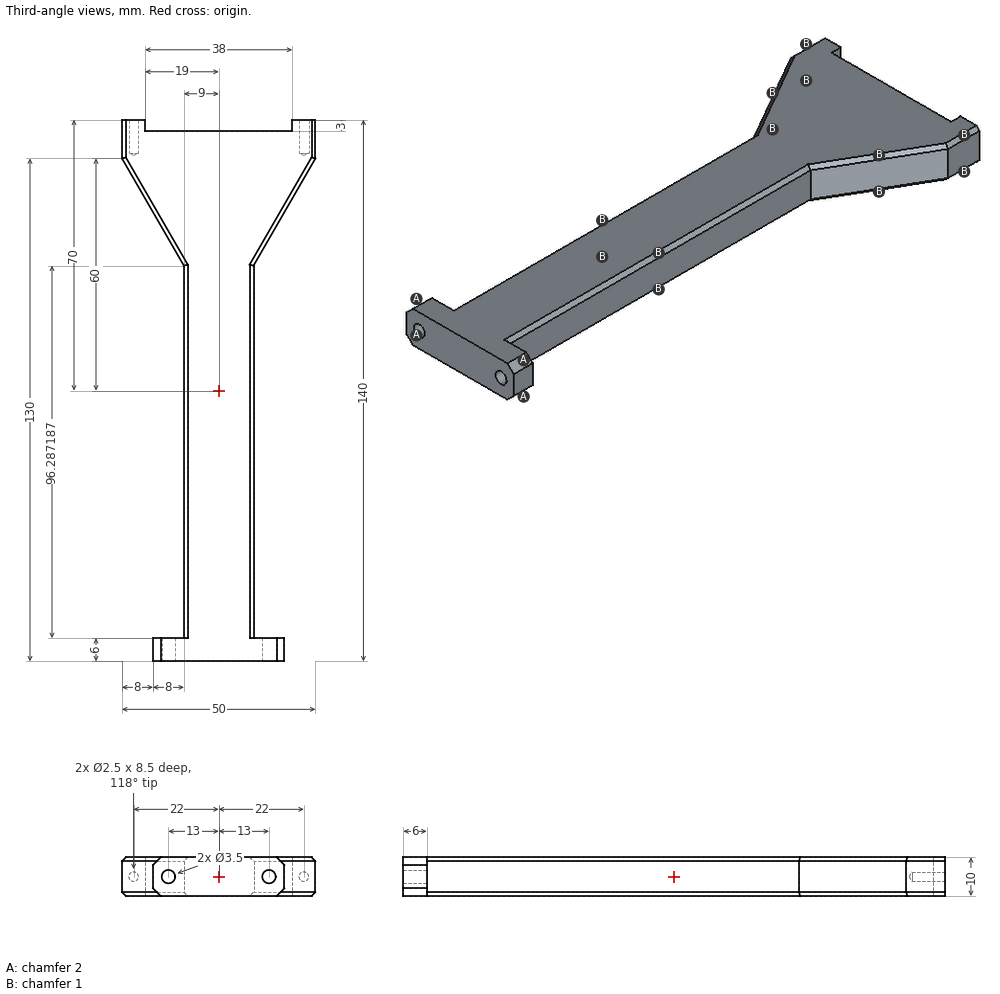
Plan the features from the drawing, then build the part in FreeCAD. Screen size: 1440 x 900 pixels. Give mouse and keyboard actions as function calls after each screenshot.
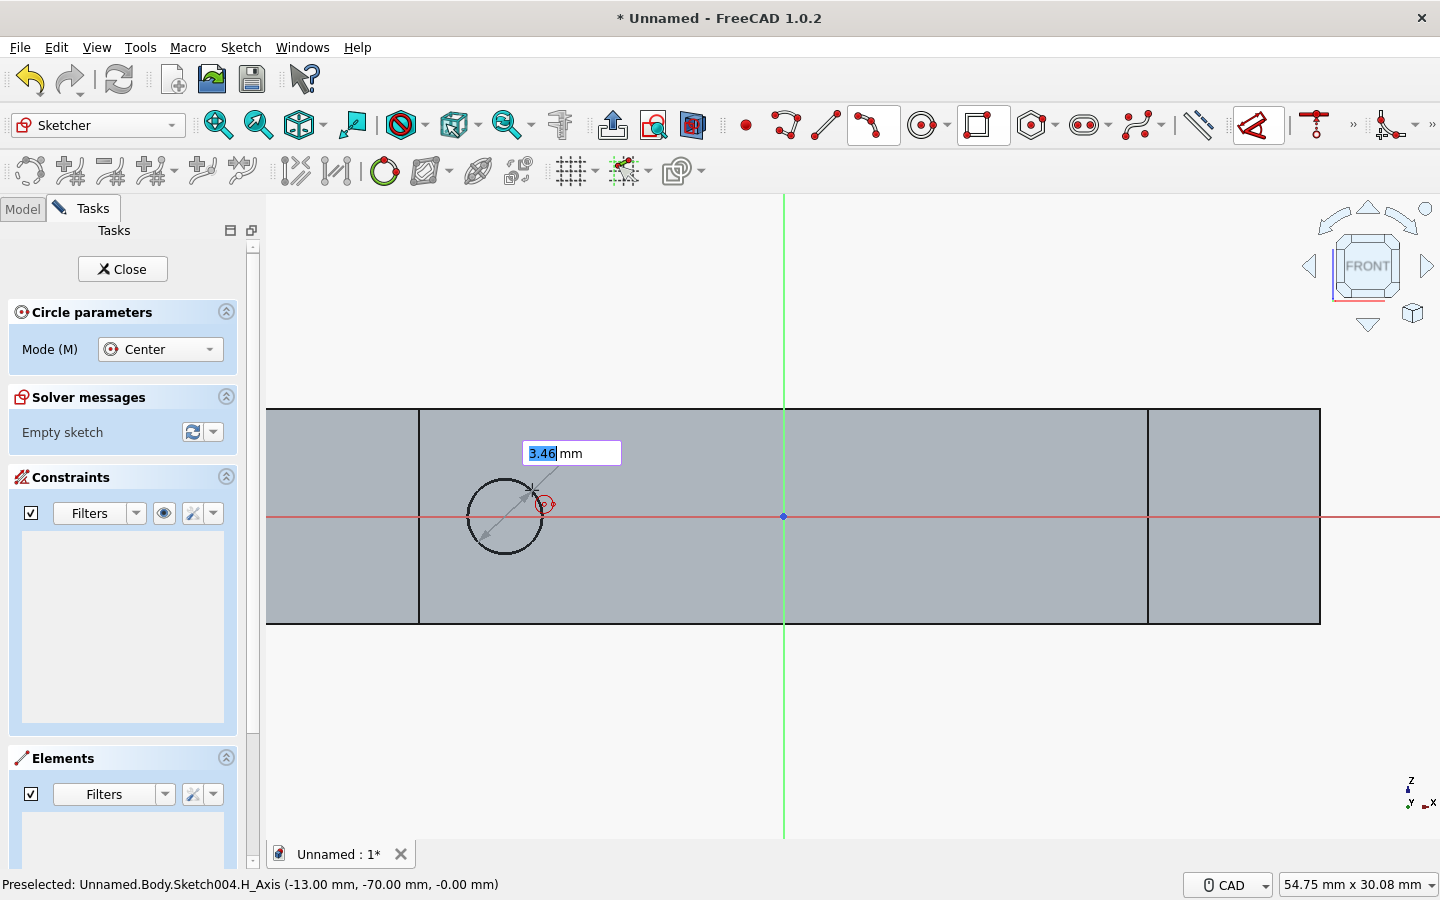
text(3.5)
key(Return)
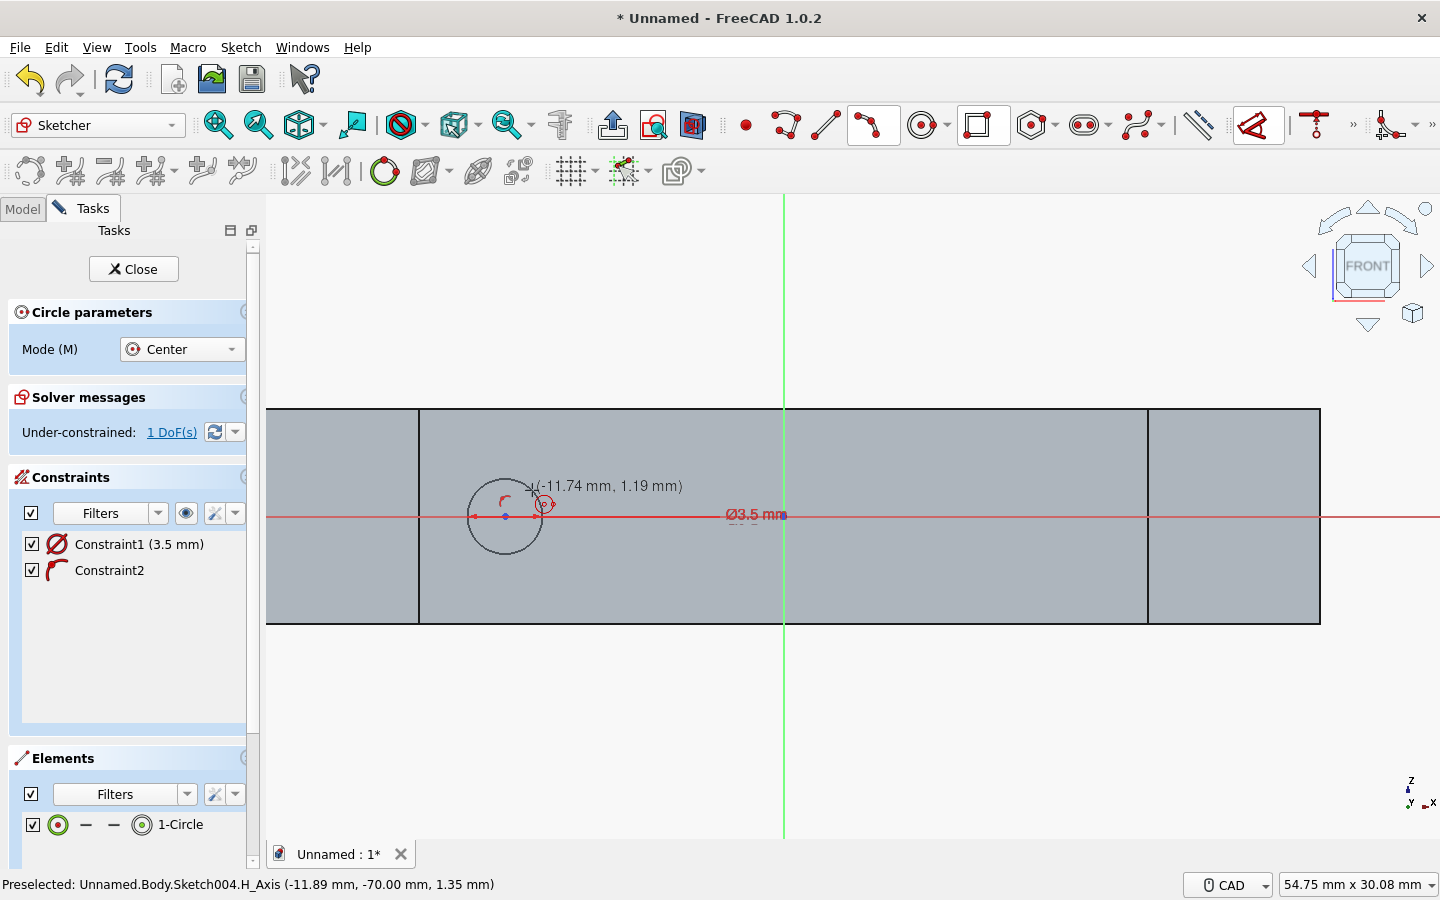
click(1063, 516)
move(1089, 490)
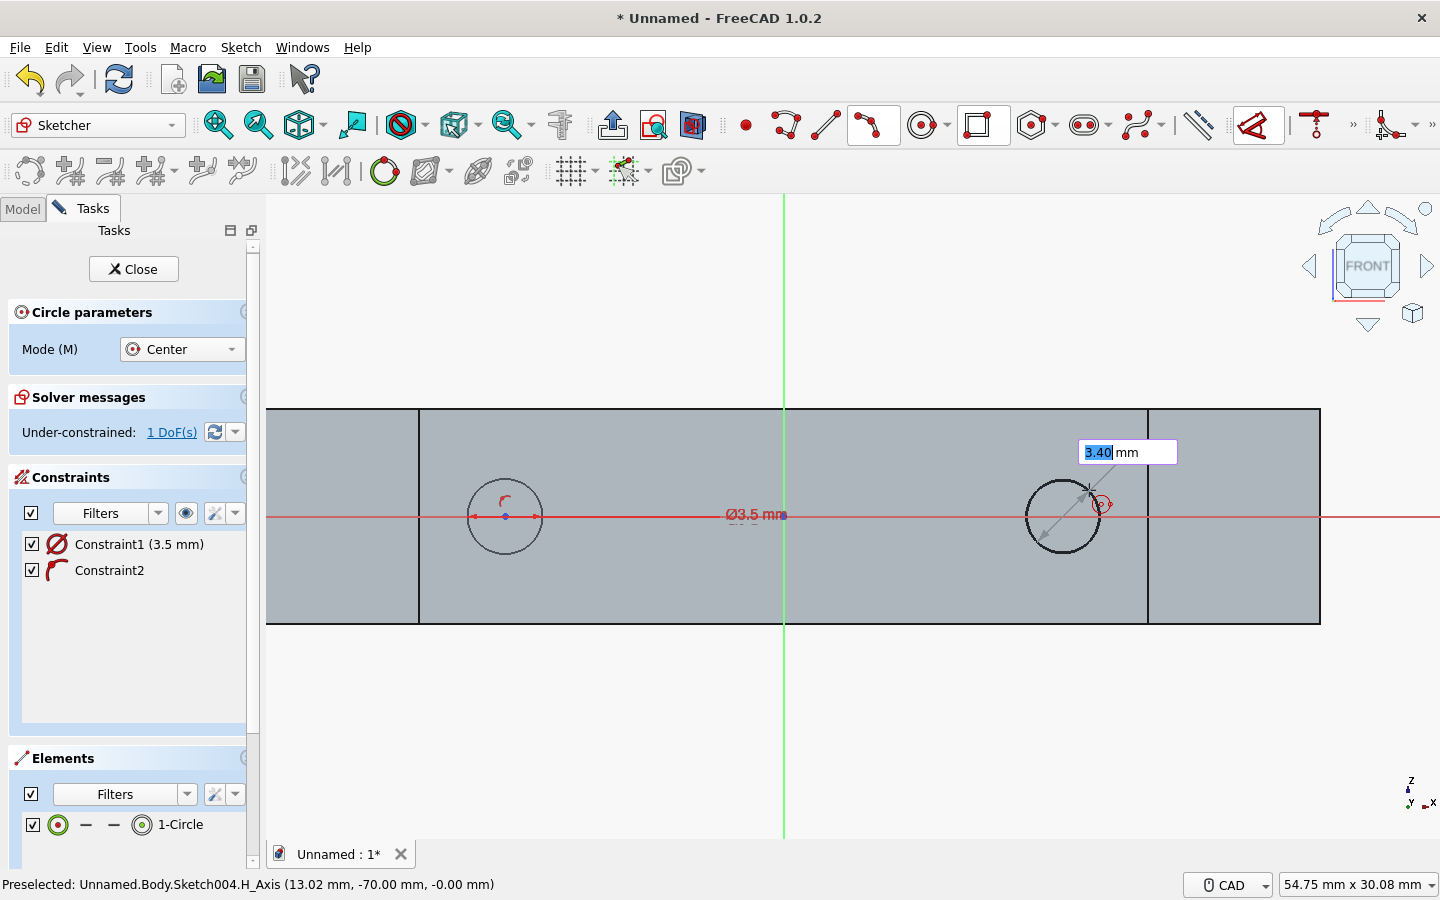
text(3.5)
key(Return)
key(Escape)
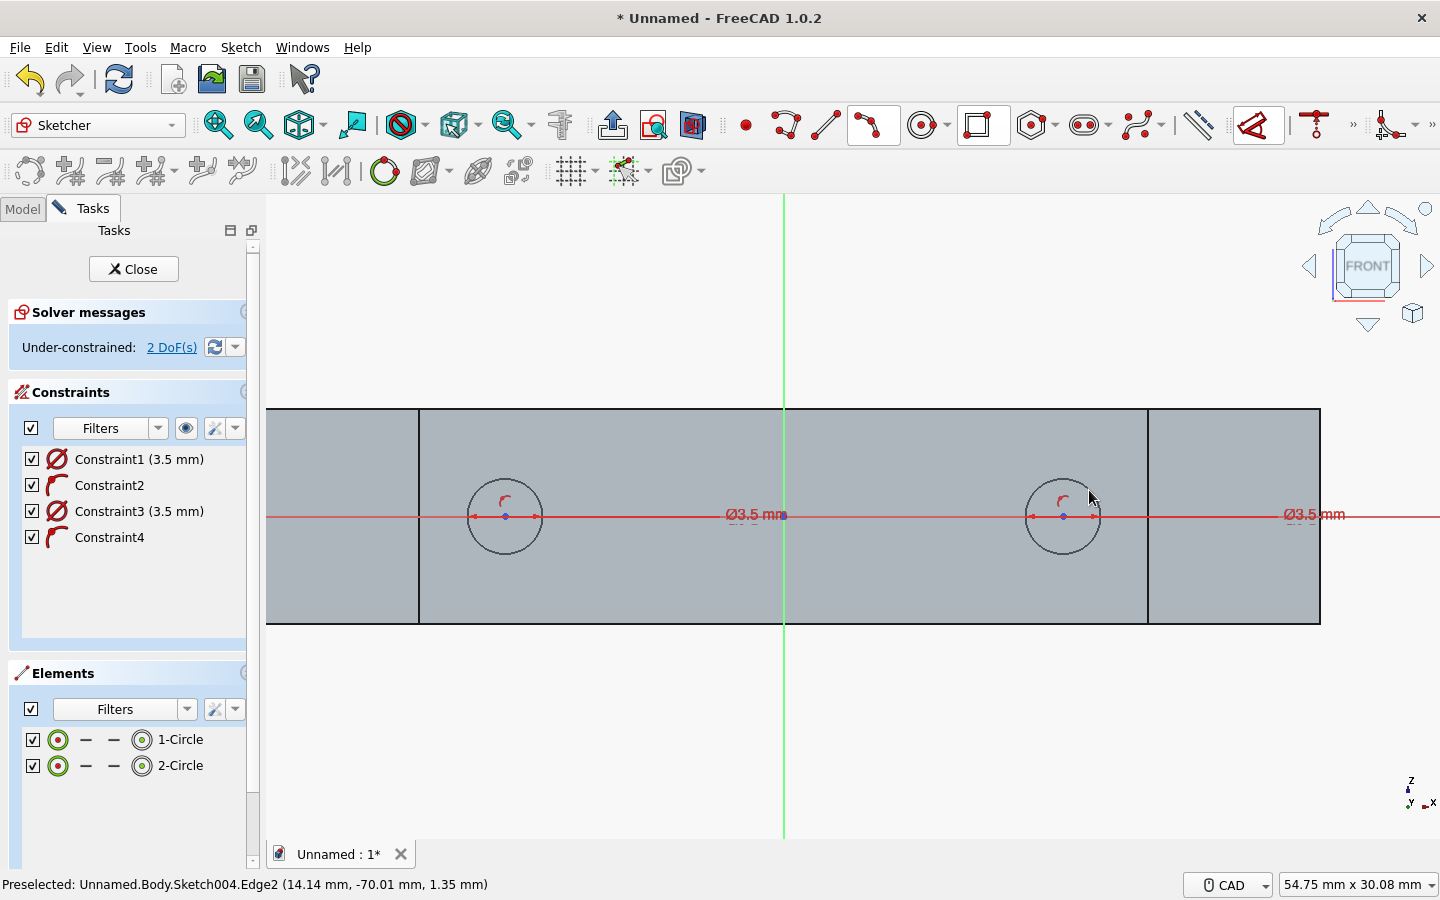
click(505, 516)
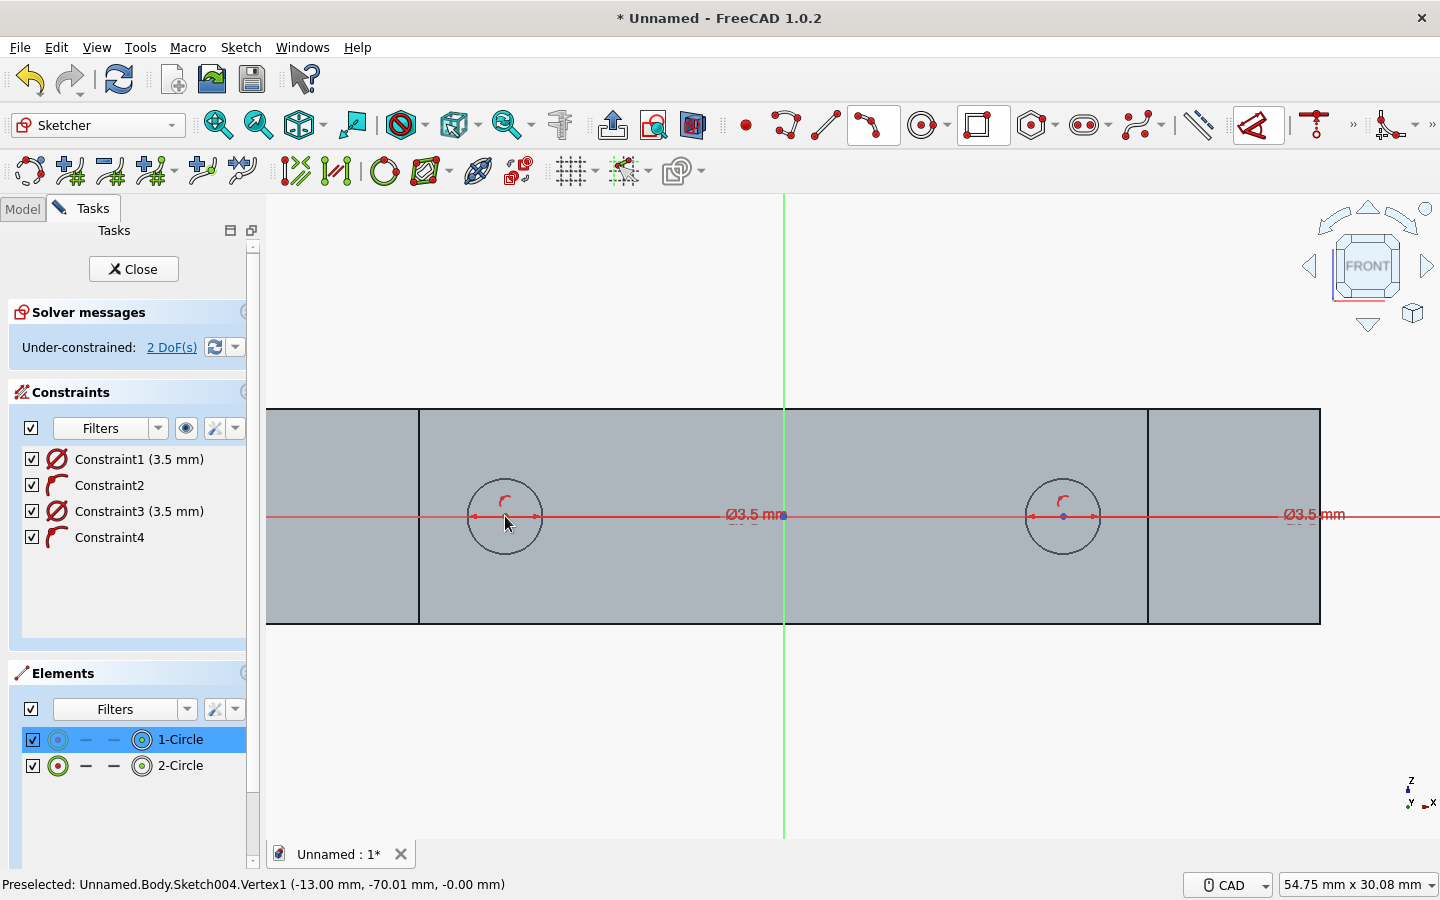
click(1278, 126)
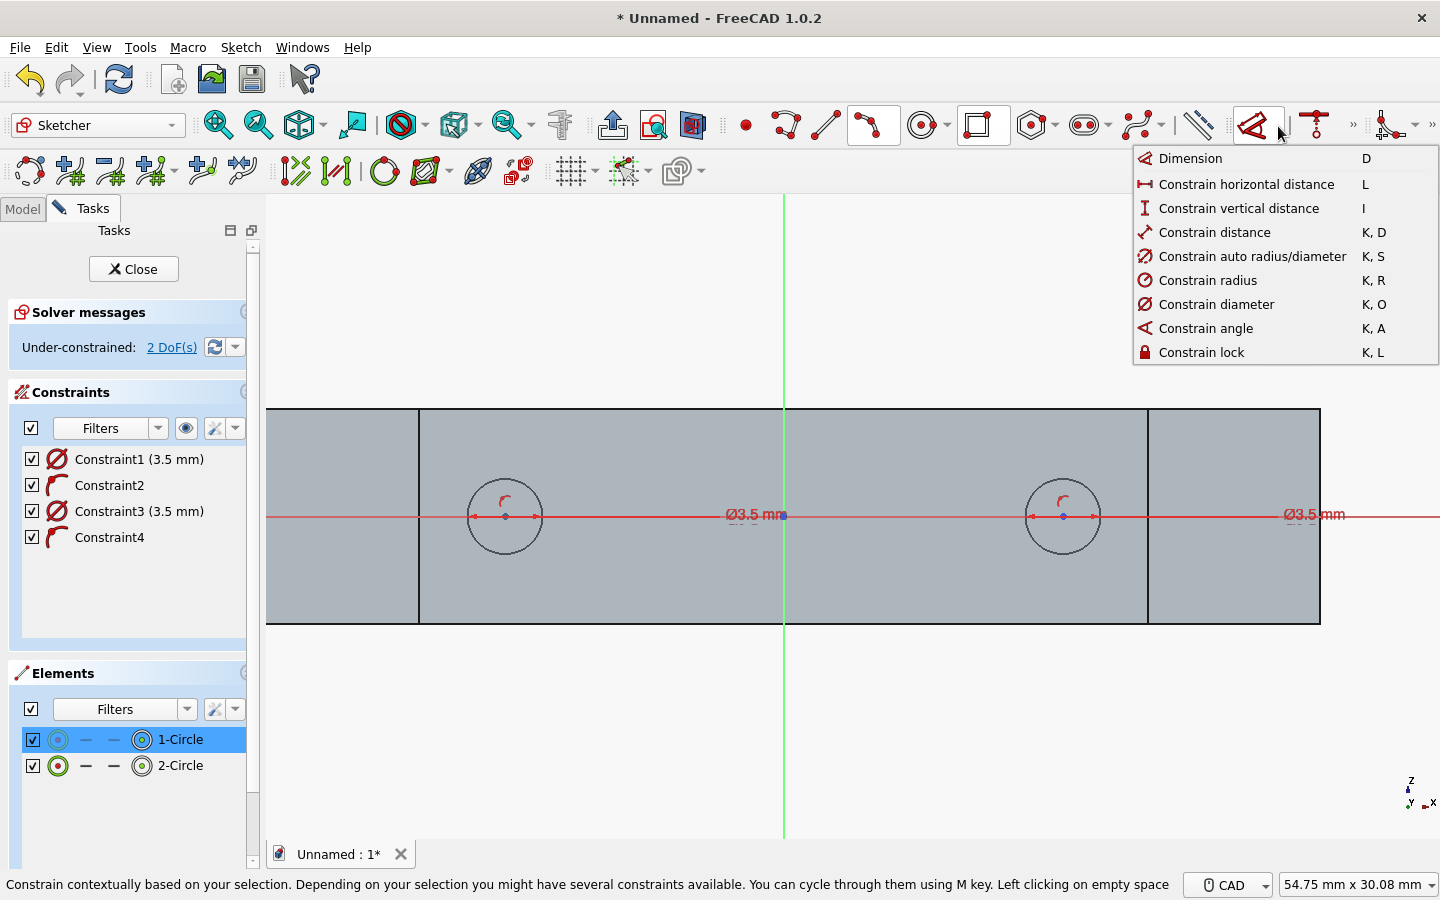
click(1286, 184)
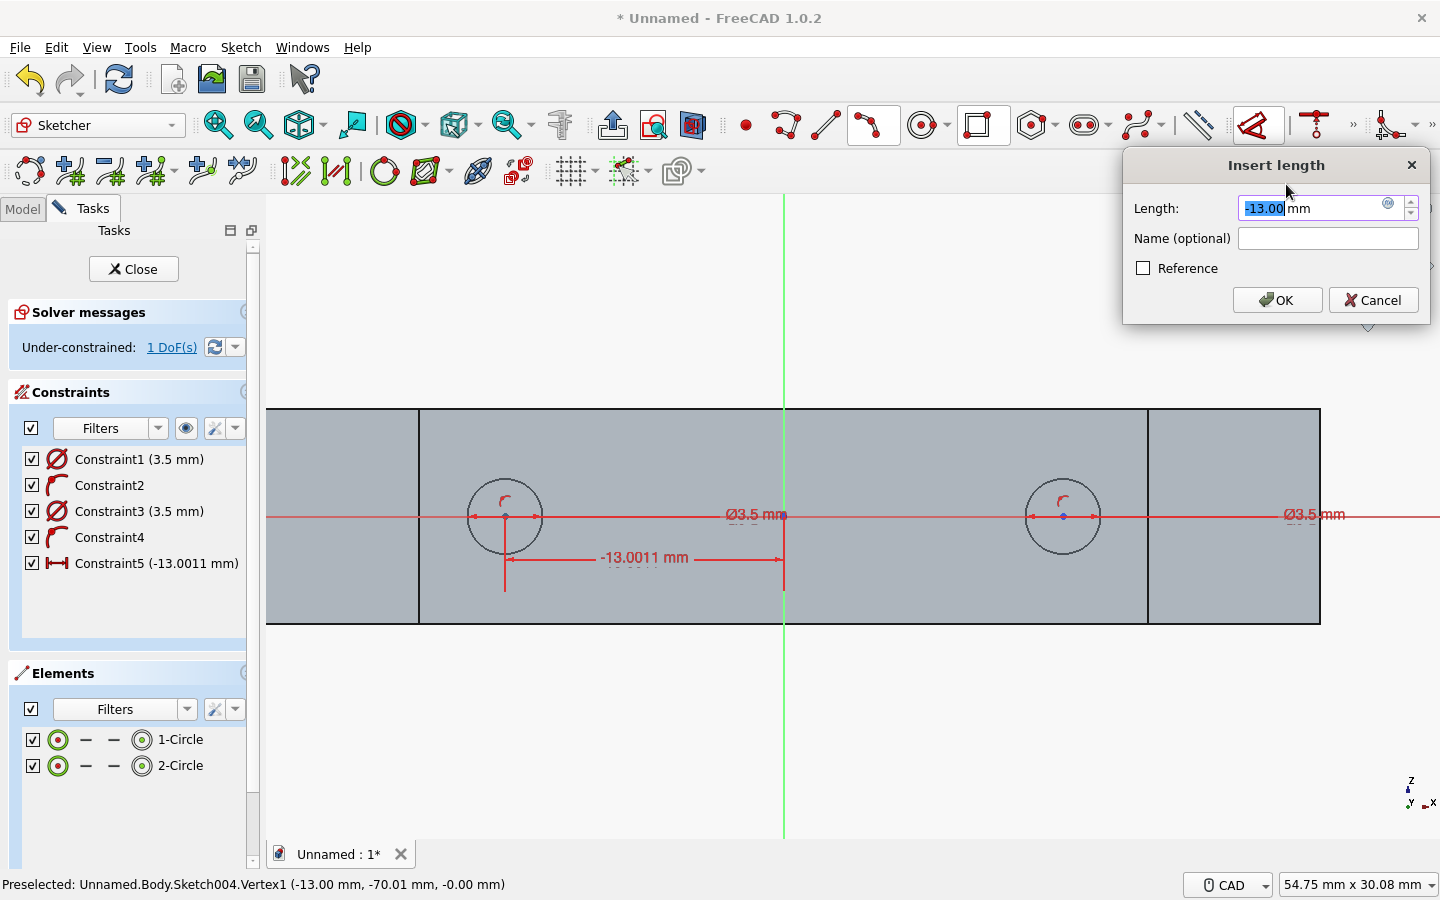
text(-13)
key(Return)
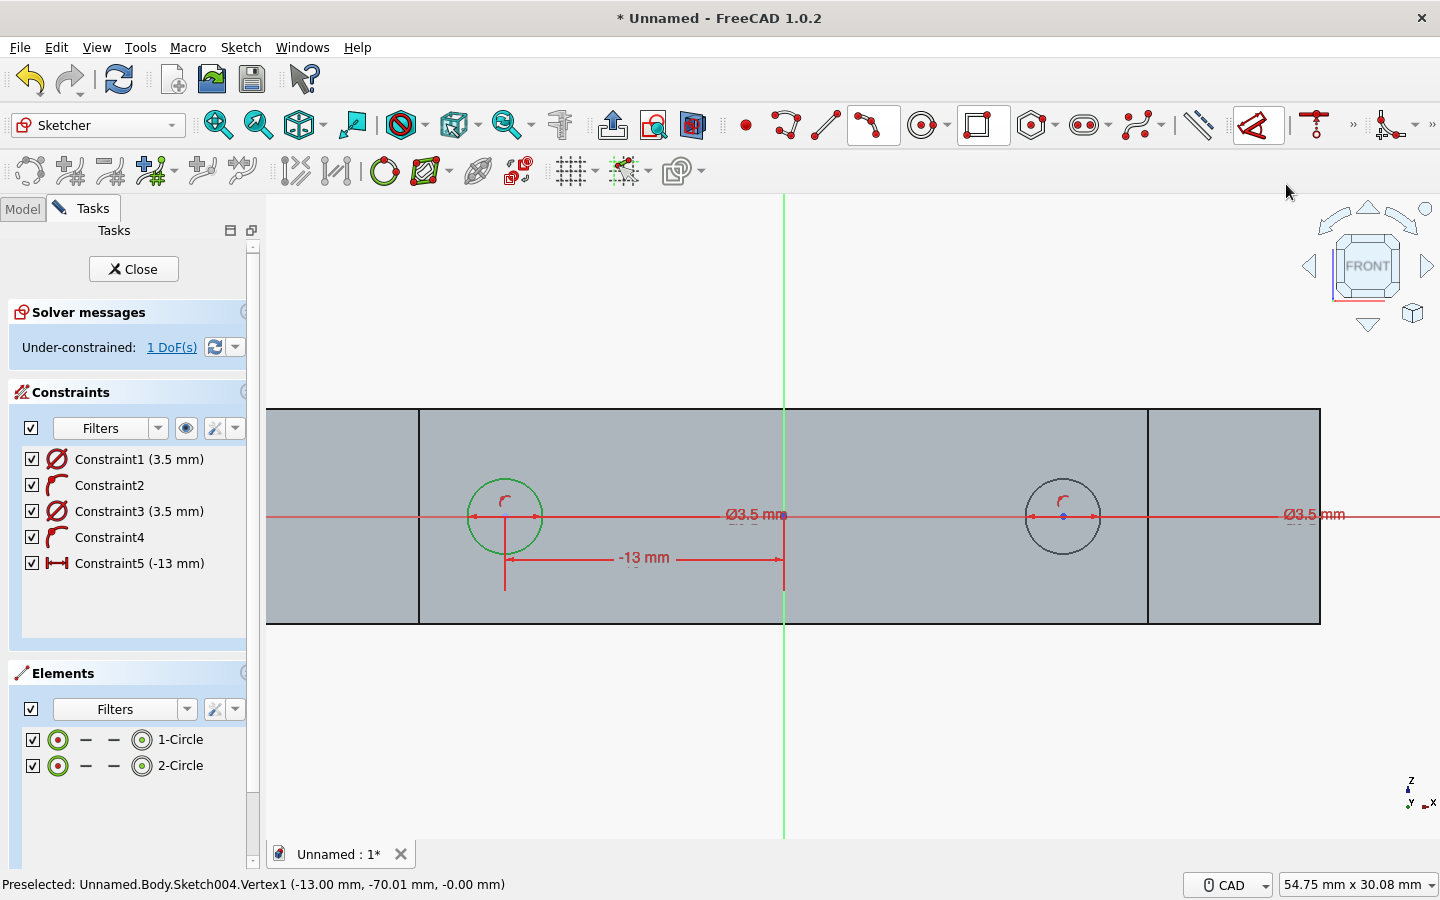
click(1063, 516)